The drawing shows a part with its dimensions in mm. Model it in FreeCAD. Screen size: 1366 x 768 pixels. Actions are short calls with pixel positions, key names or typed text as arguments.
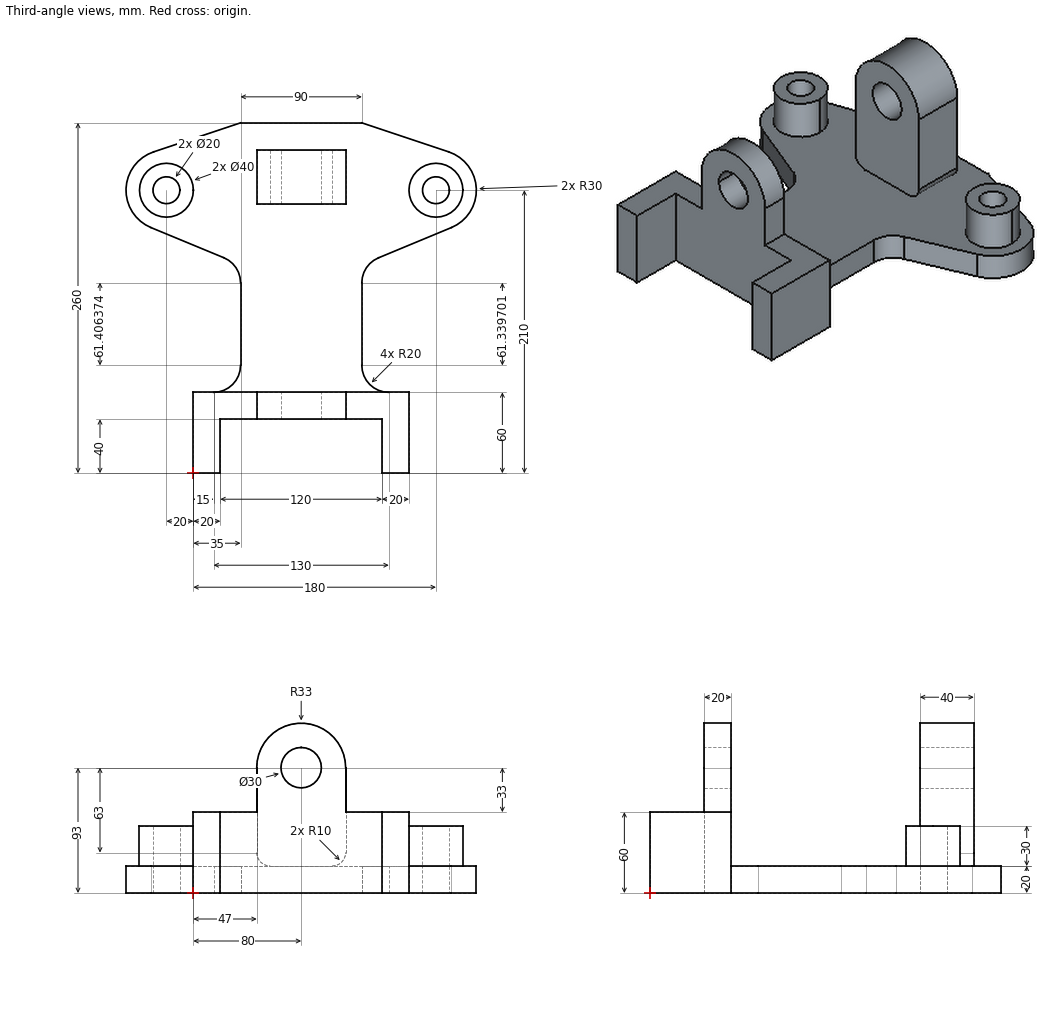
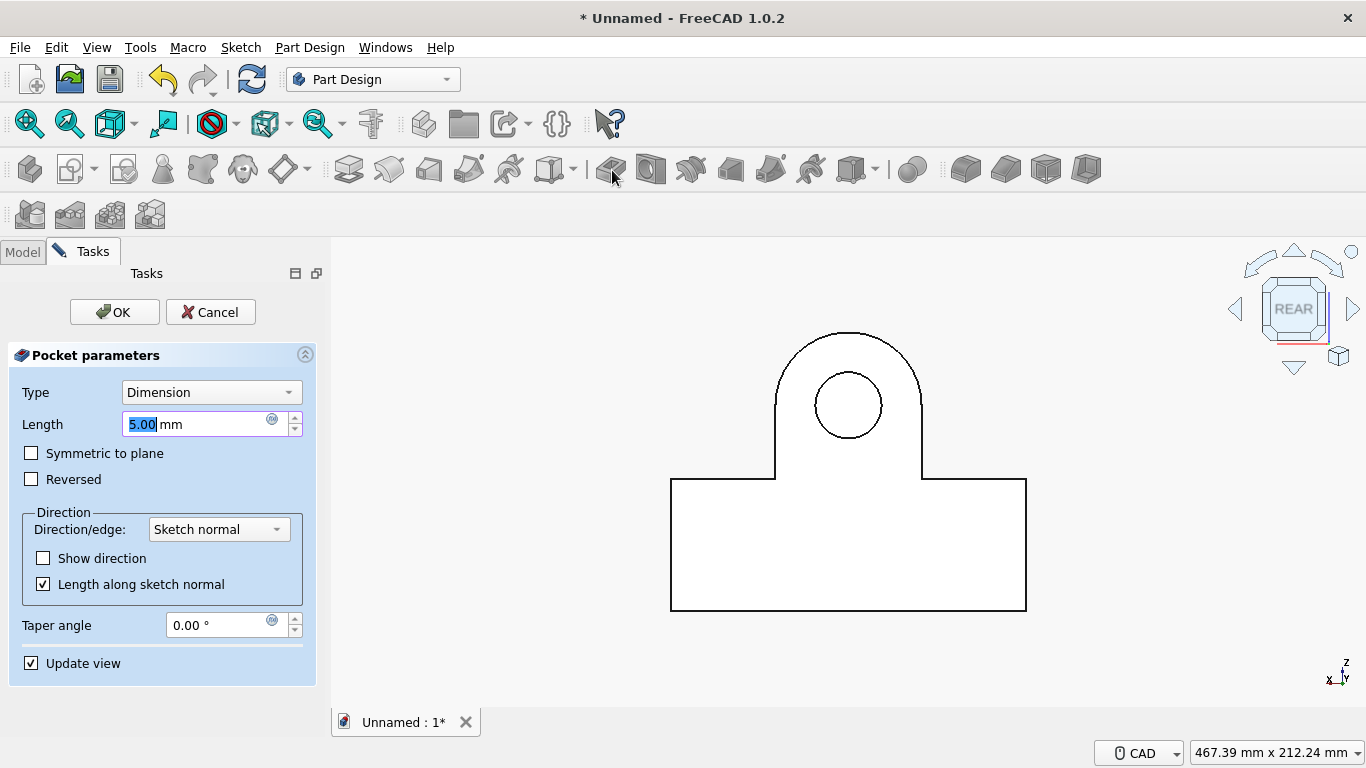
text(20)
key(Tab)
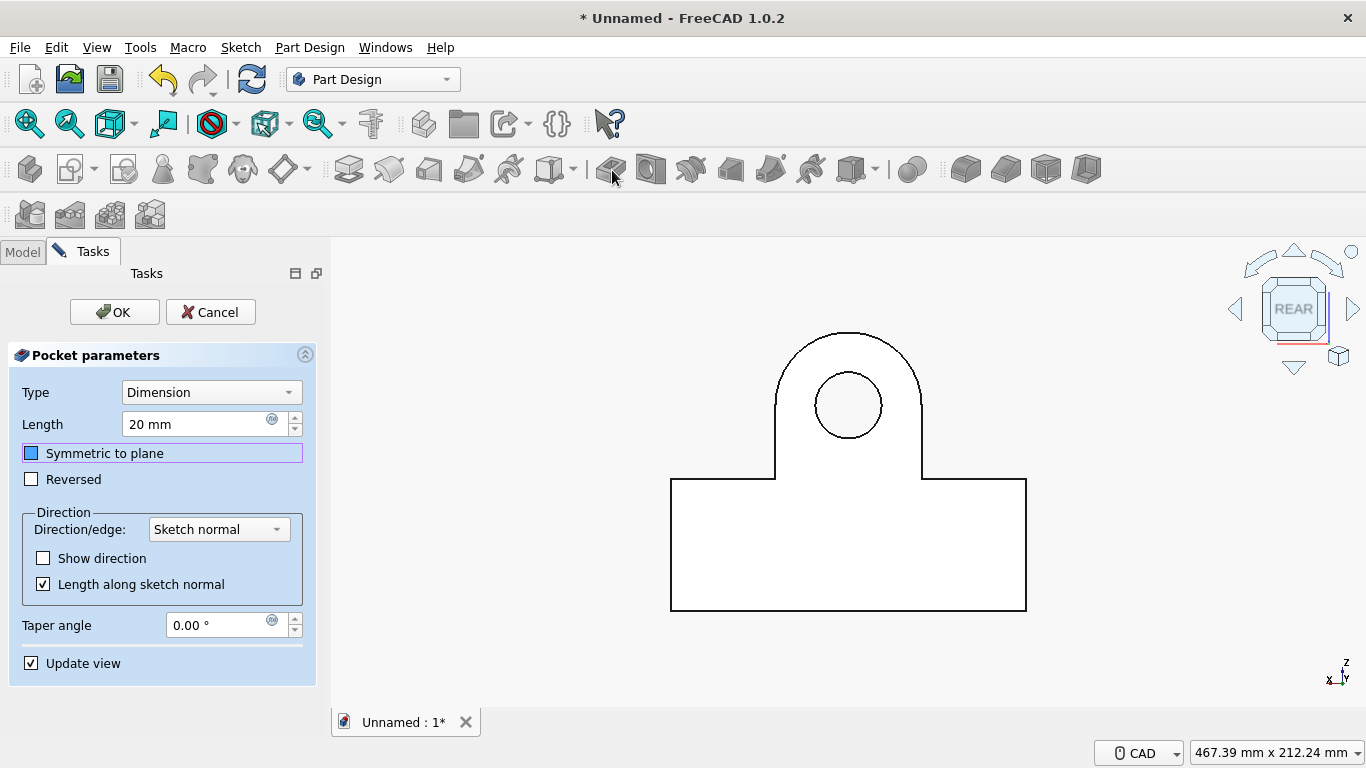
click(115, 312)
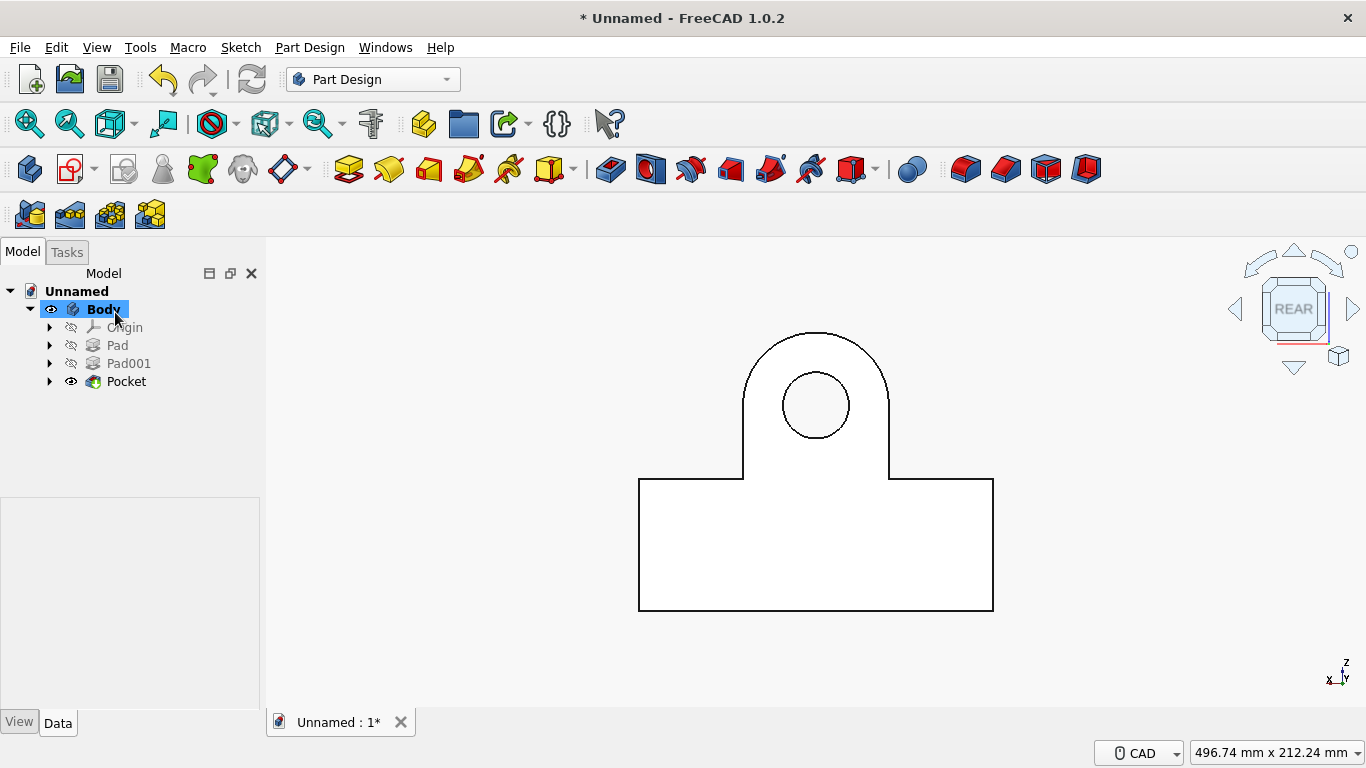
key(5)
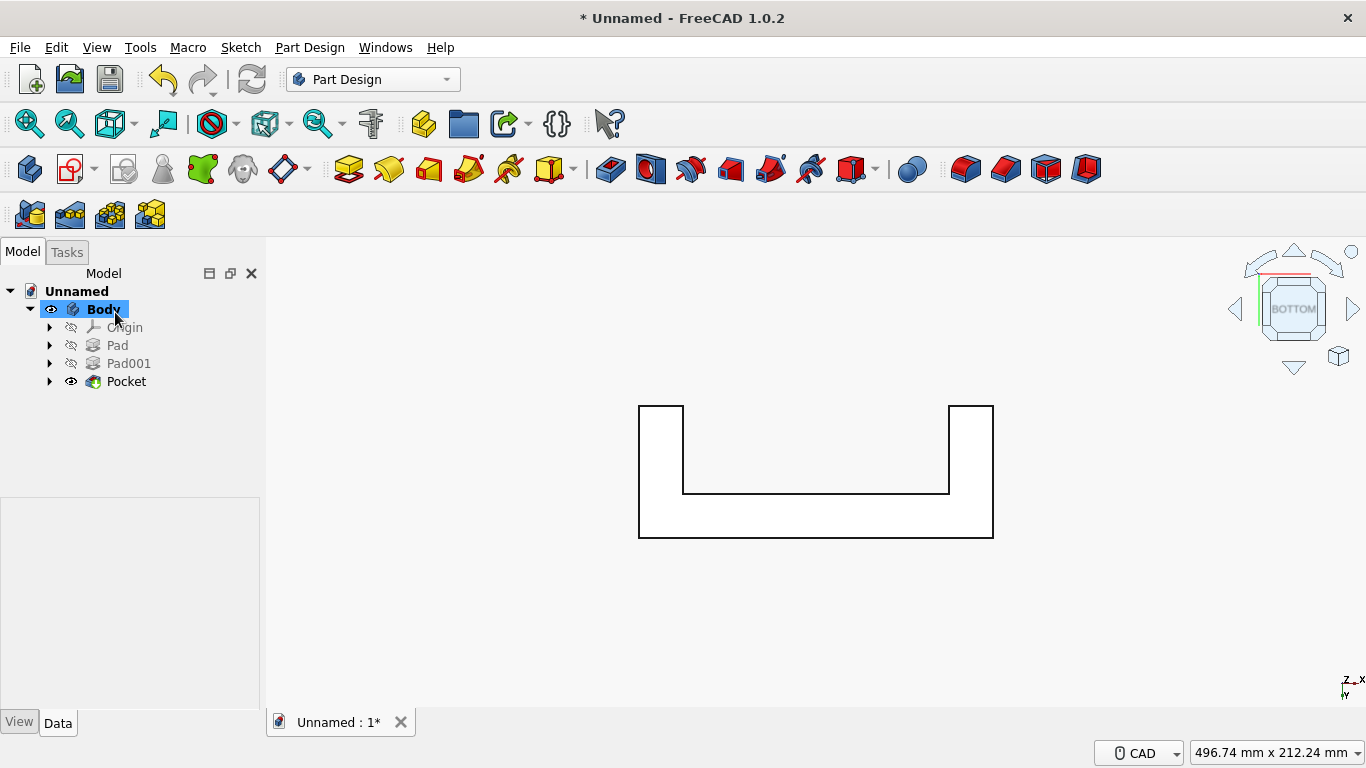
click(30, 124)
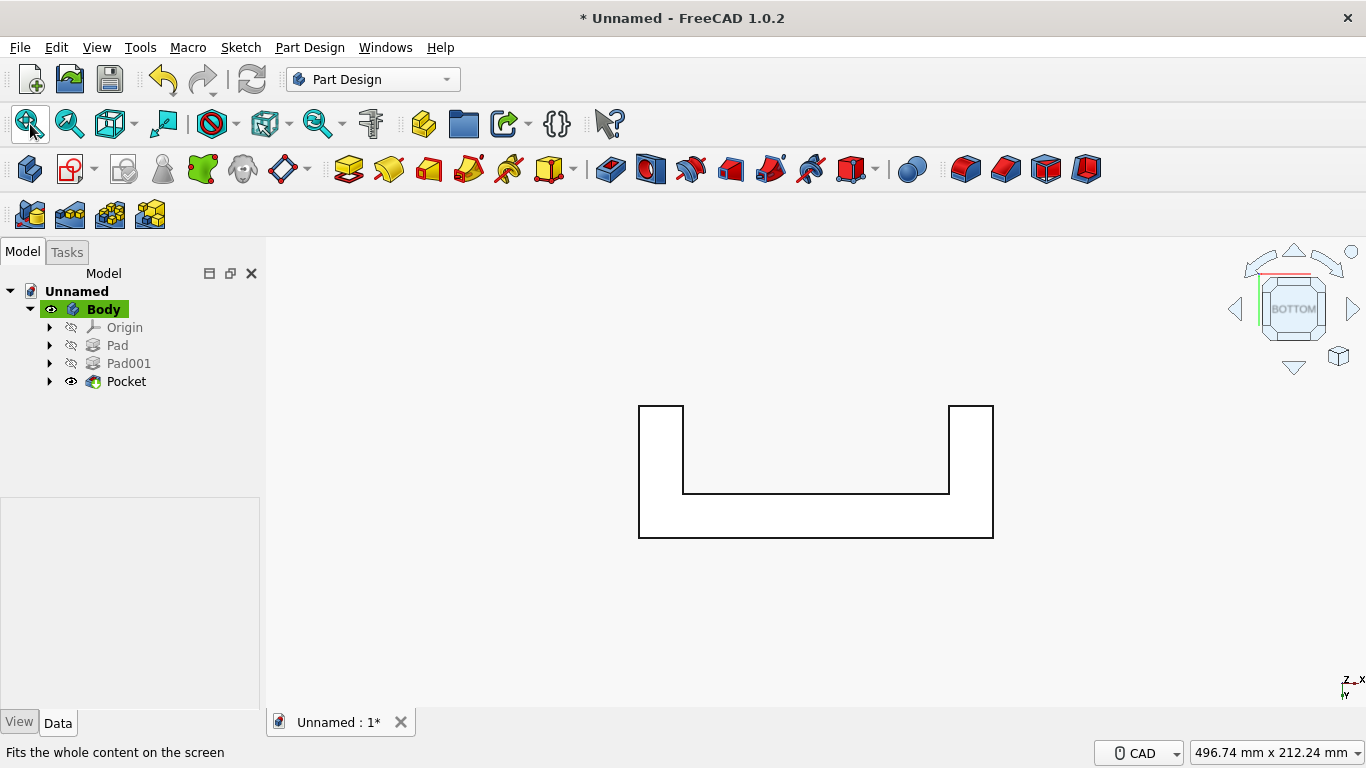
click(968, 509)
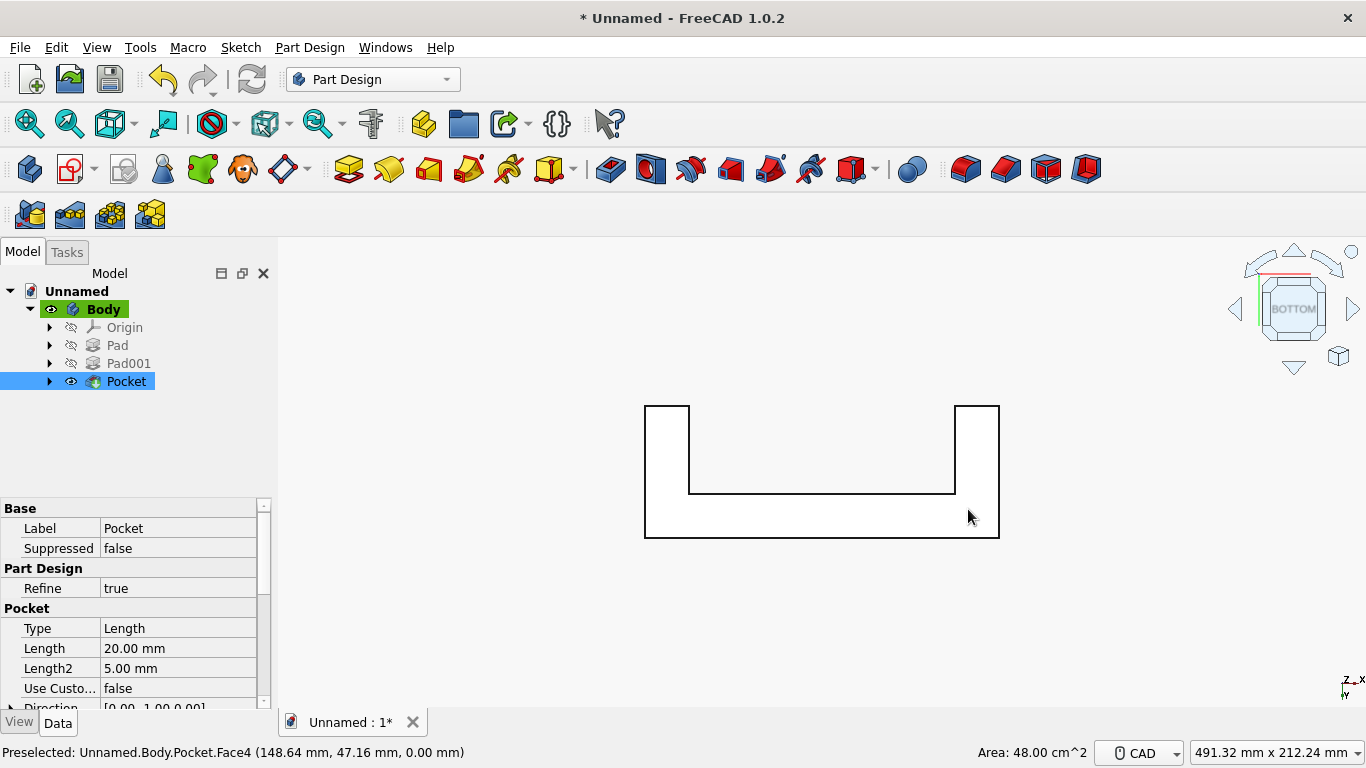
click(70, 170)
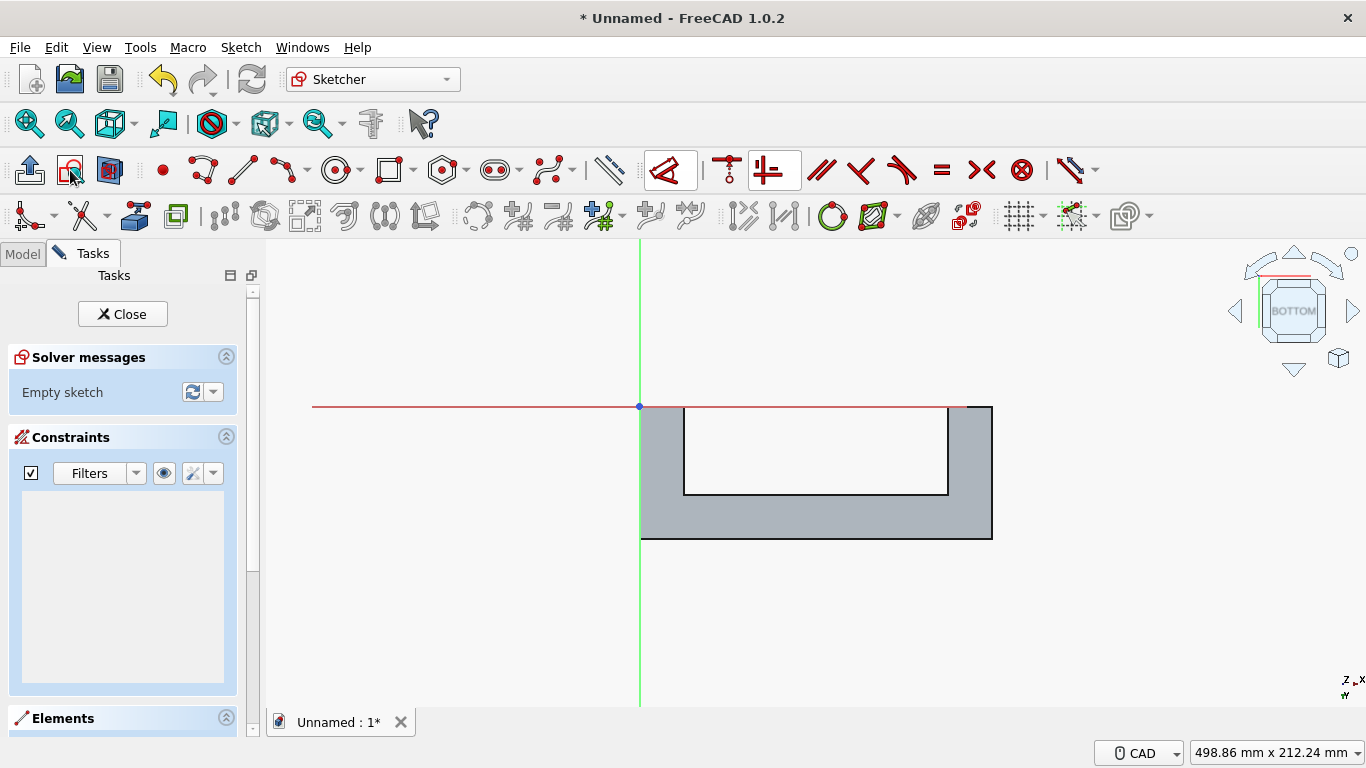
scroll(692, 293, down, 4)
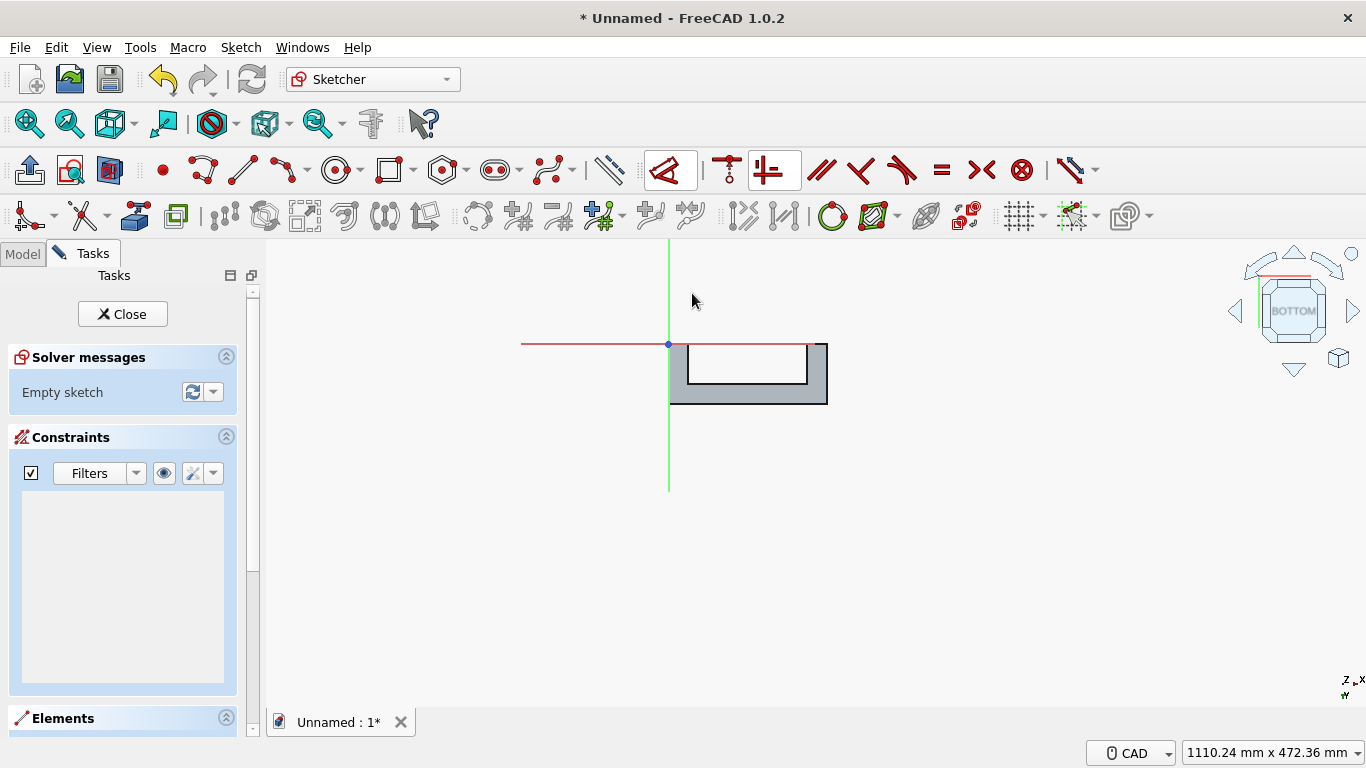
key(g)
key(l)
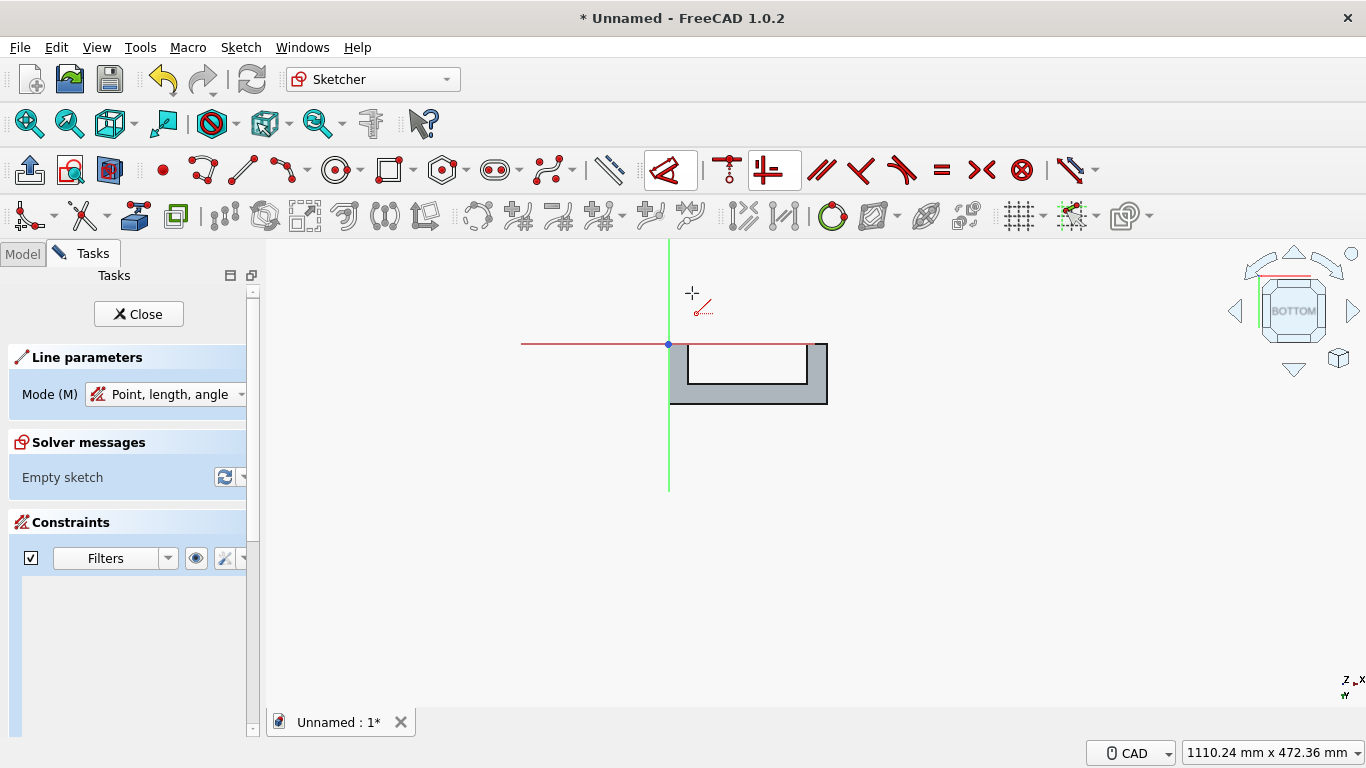
click(684, 404)
click(812, 404)